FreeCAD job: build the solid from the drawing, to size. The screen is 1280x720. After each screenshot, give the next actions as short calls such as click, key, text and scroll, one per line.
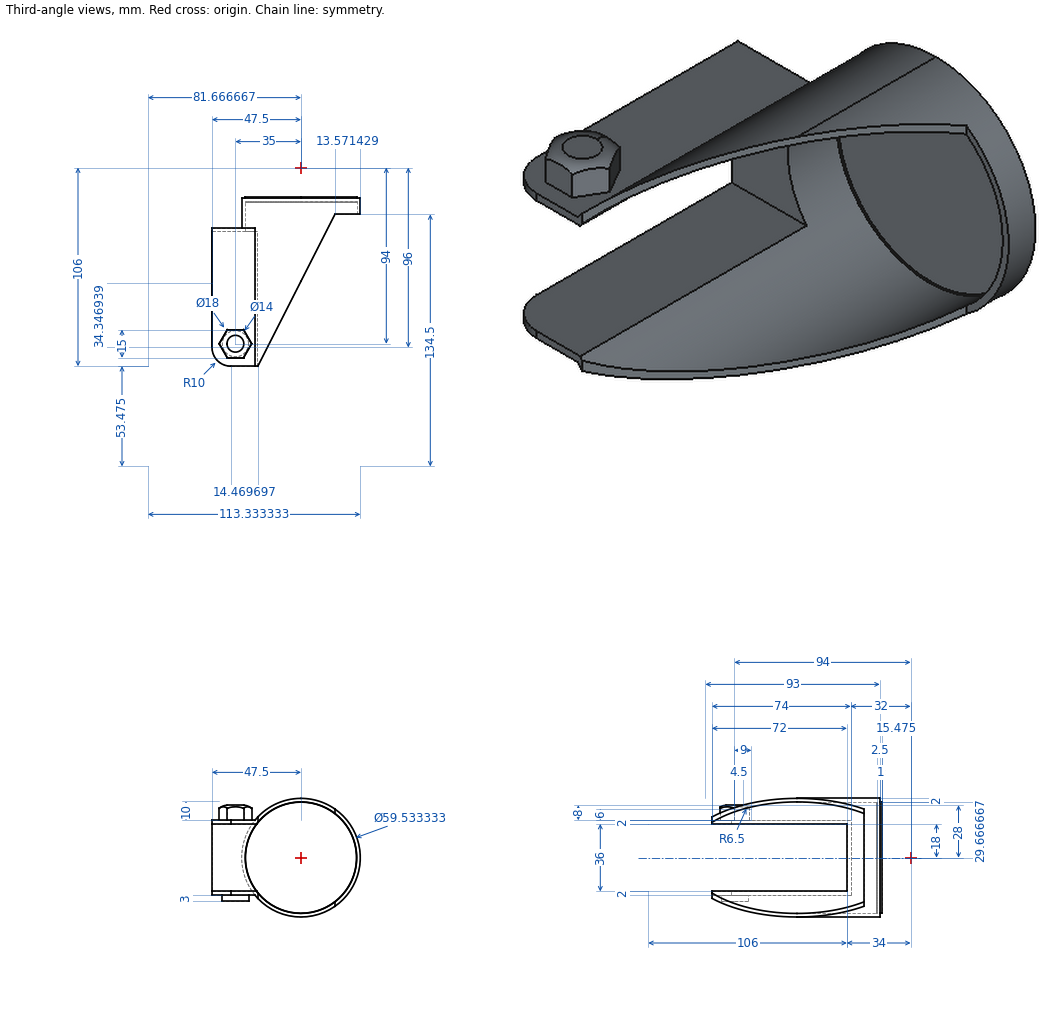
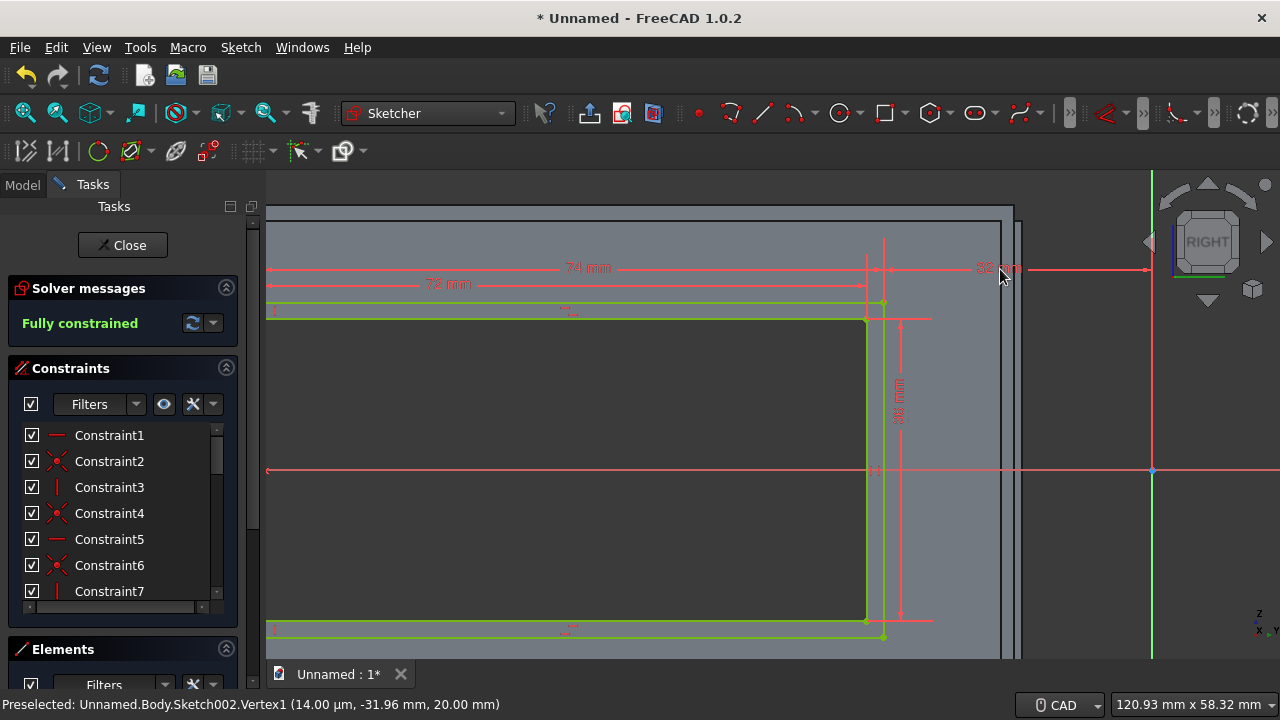
click(123, 245)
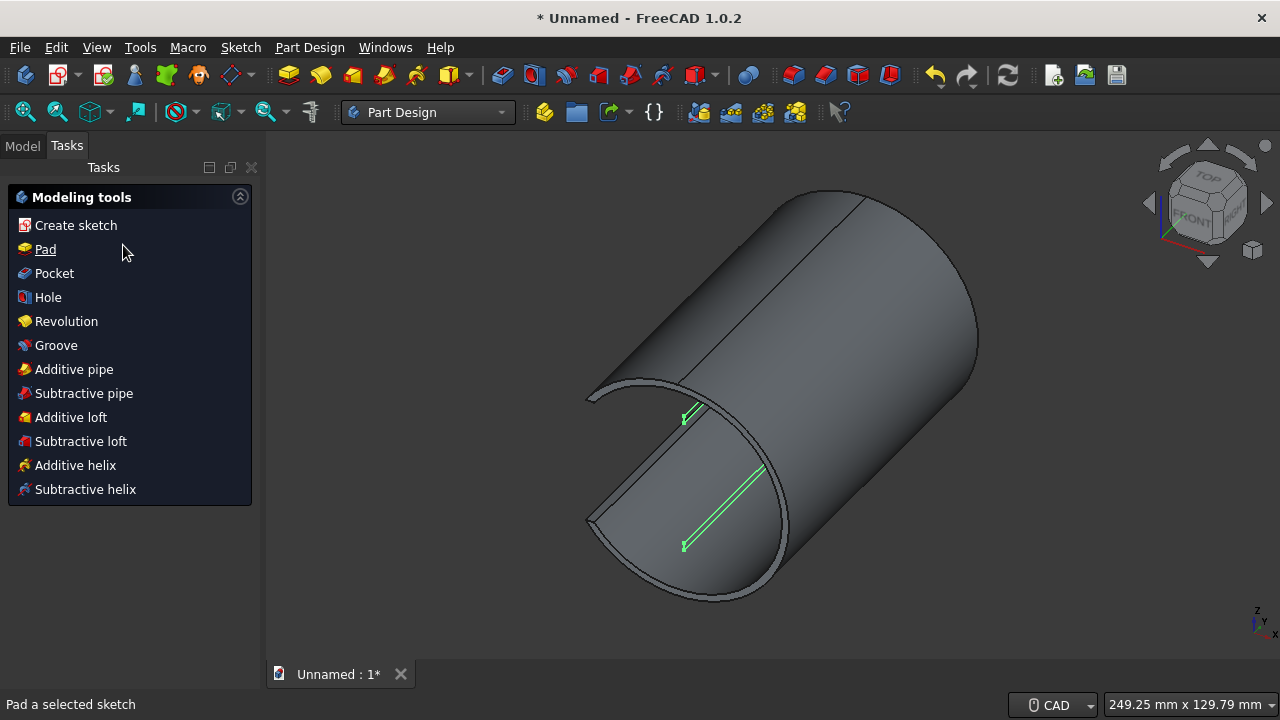
click(290, 76)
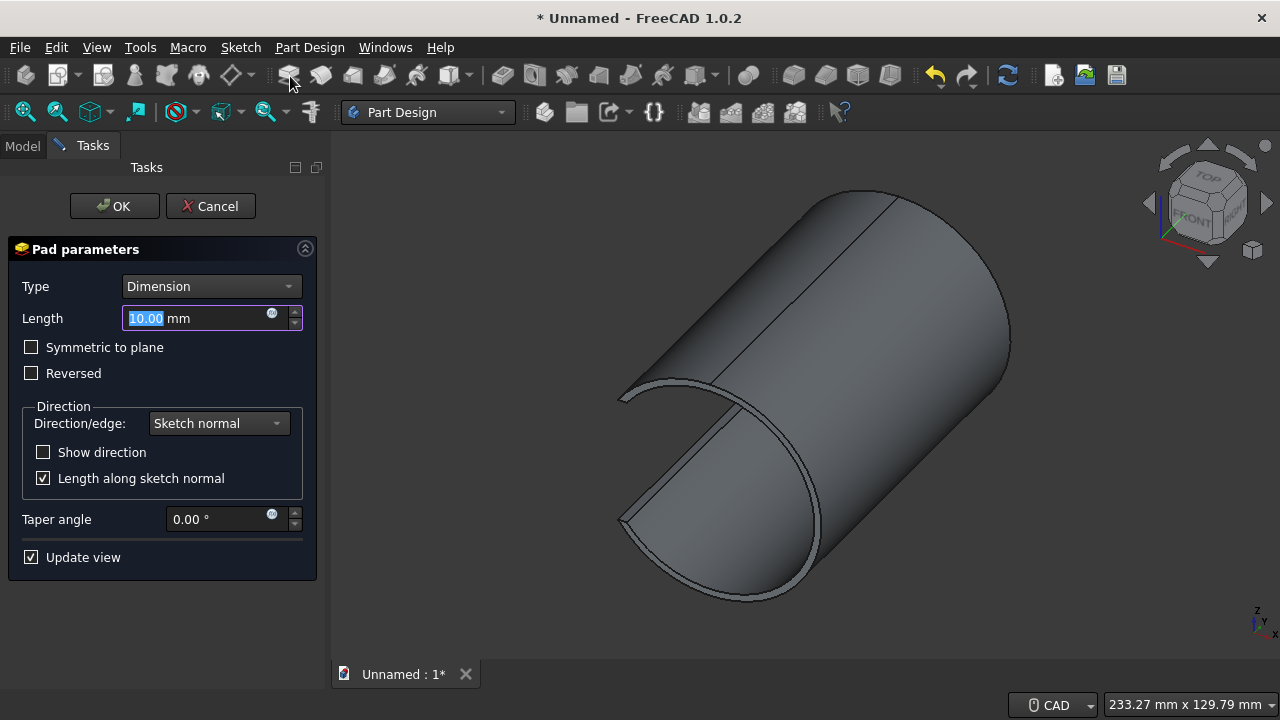
text(47.5)
key(Tab)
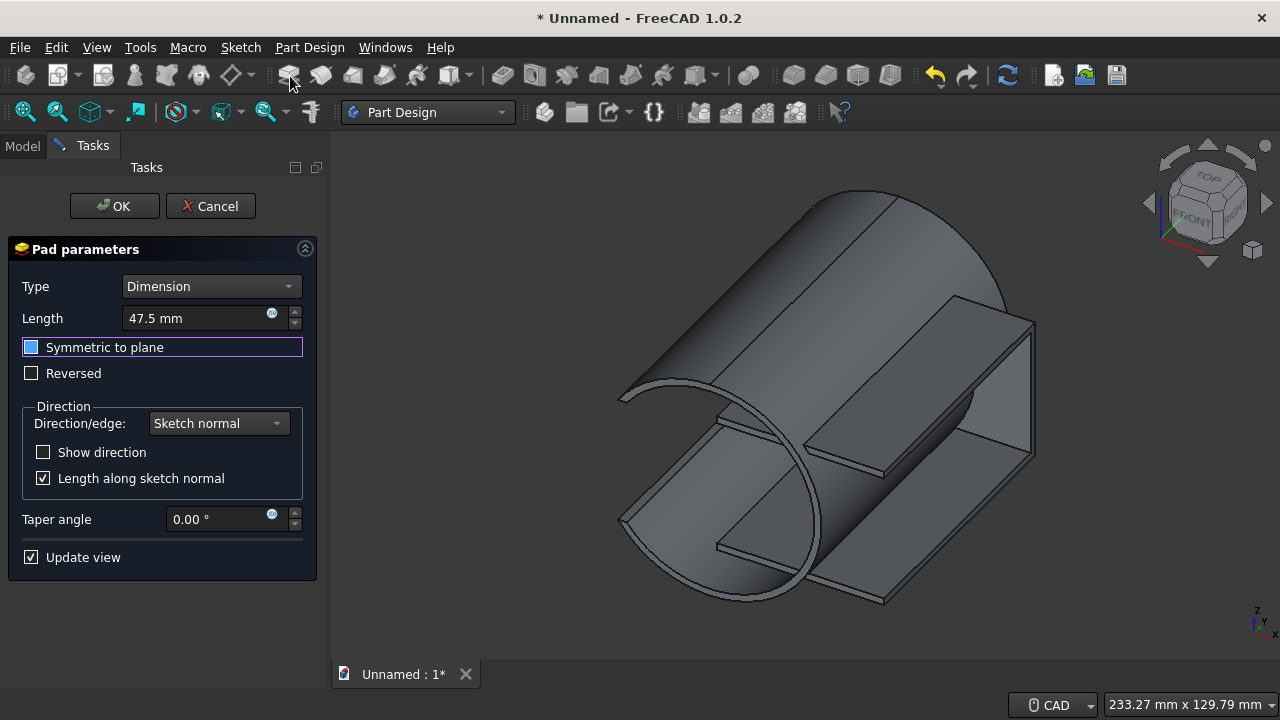
click(30, 373)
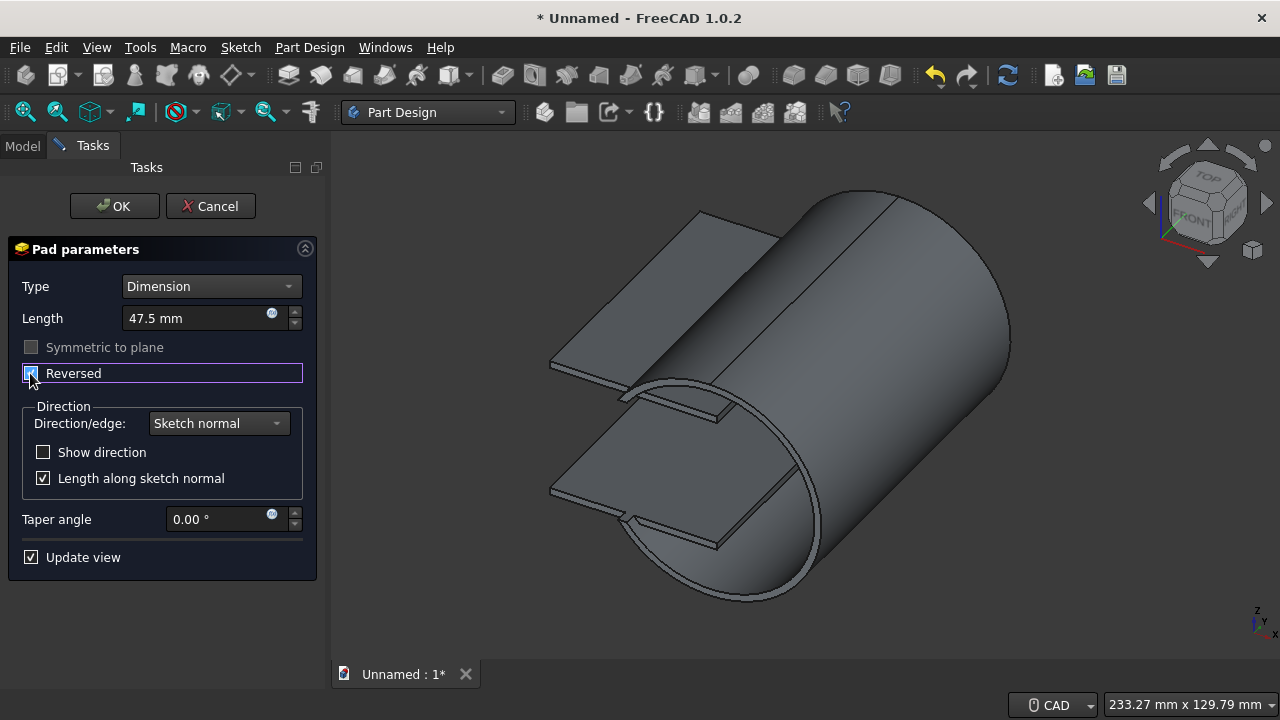
click(115, 206)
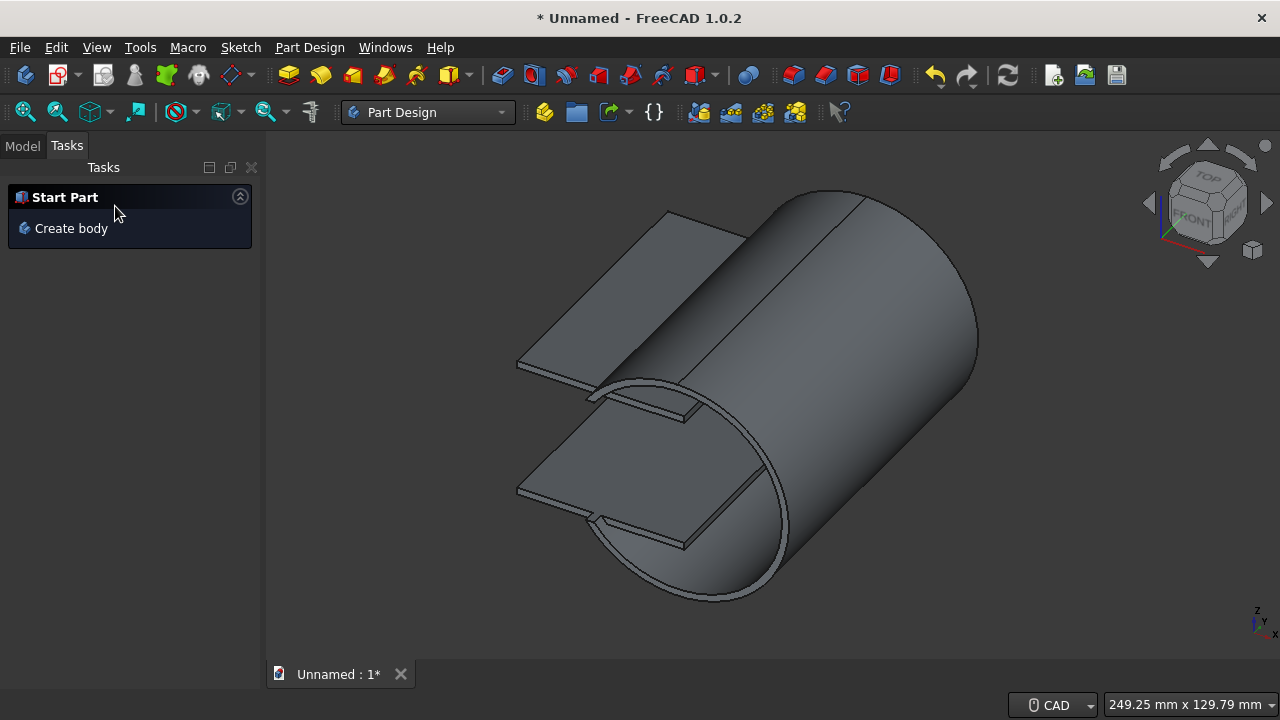
click(23, 145)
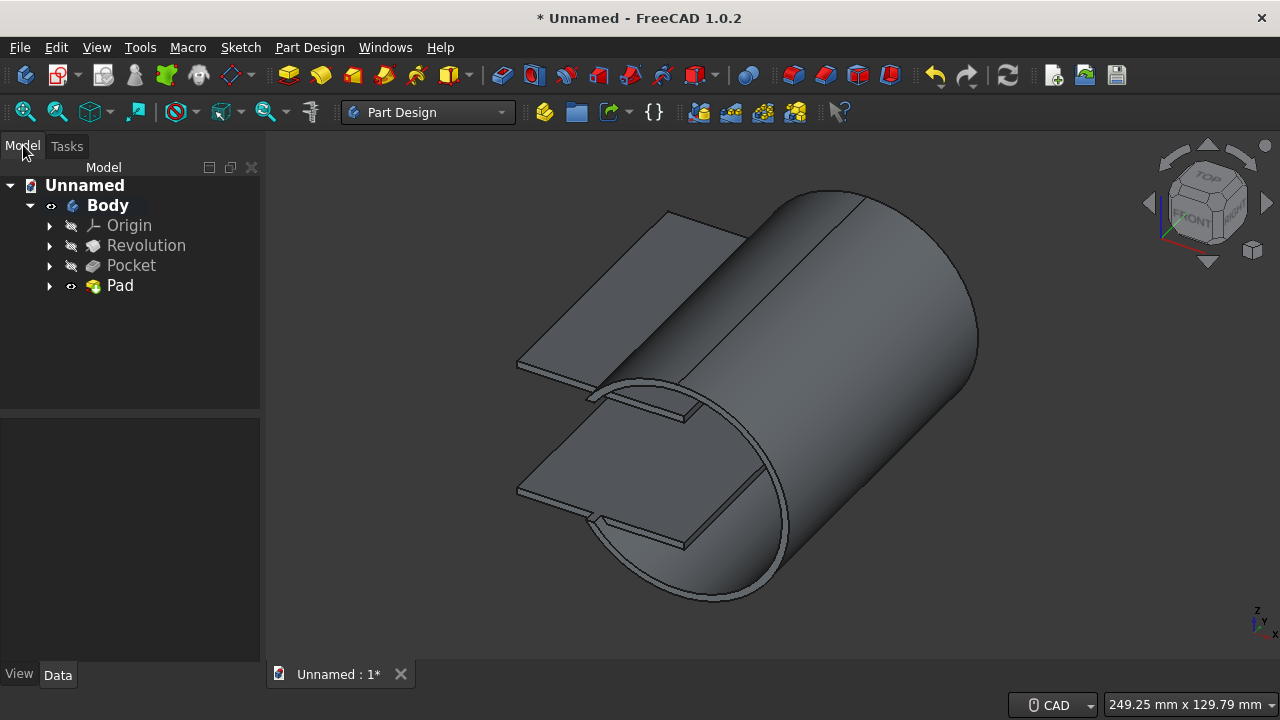
click(50, 226)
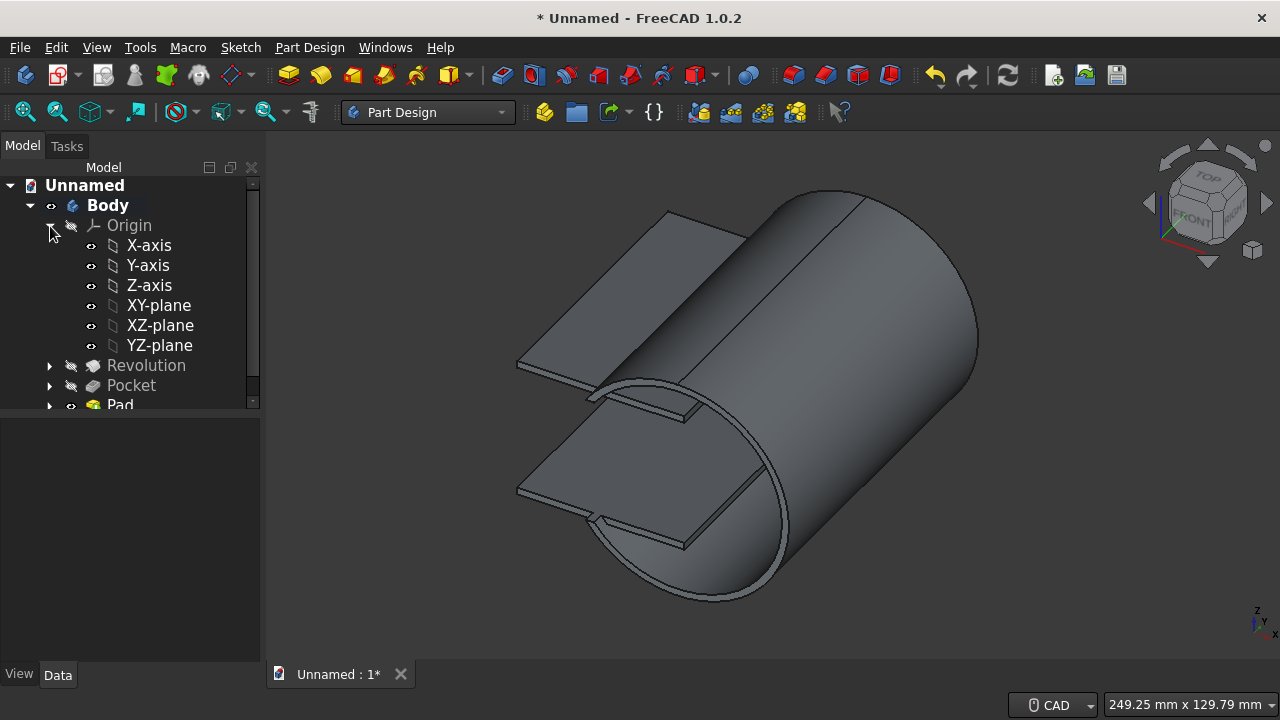
click(136, 326)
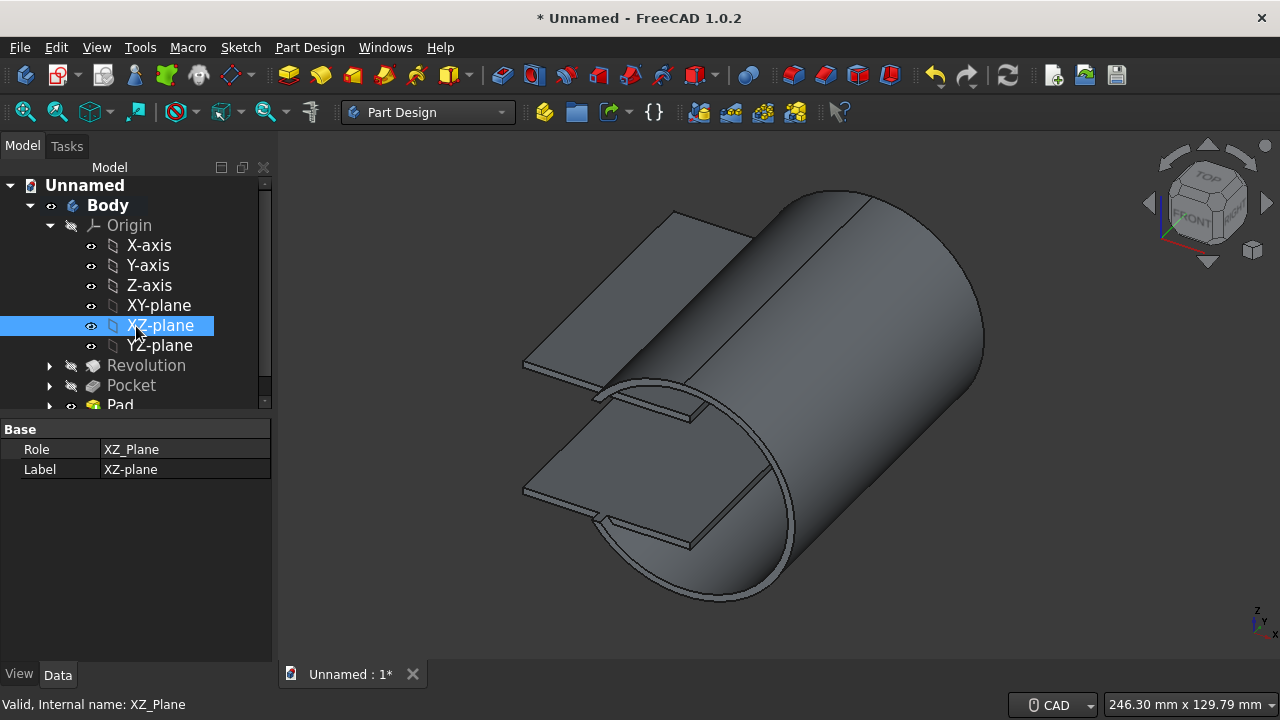
click(232, 76)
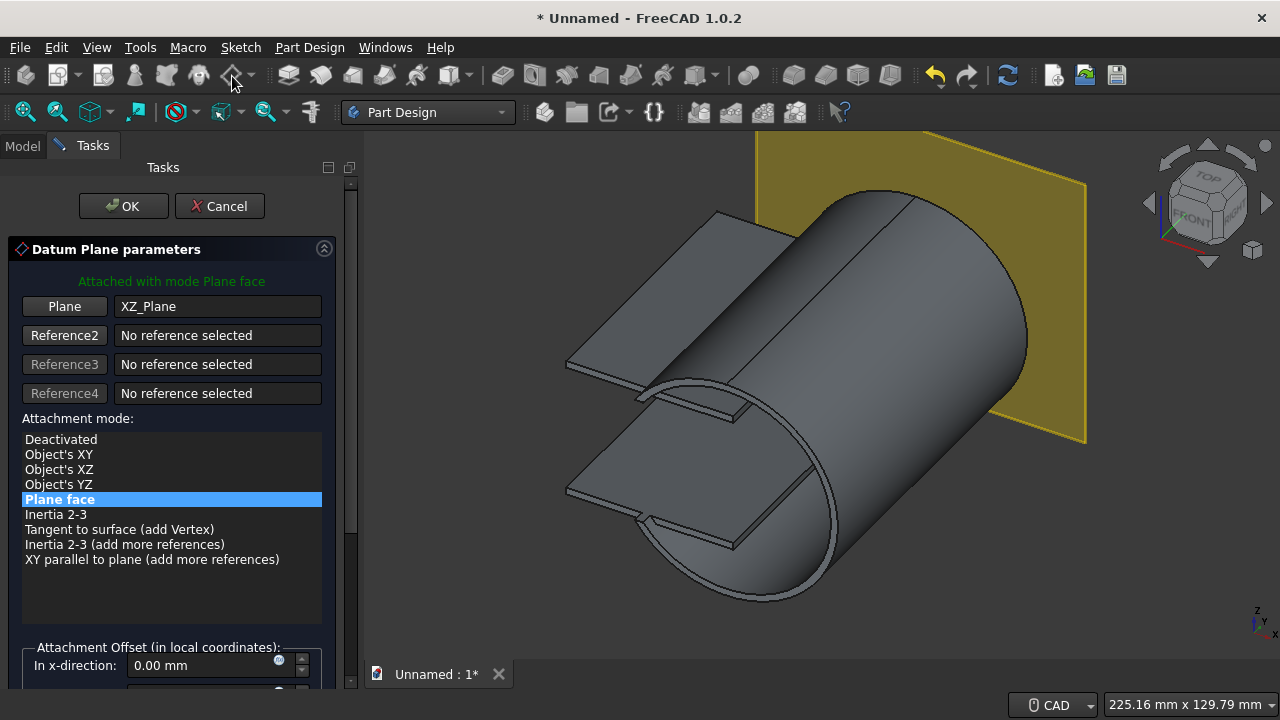
scroll(351, 432, down, 2)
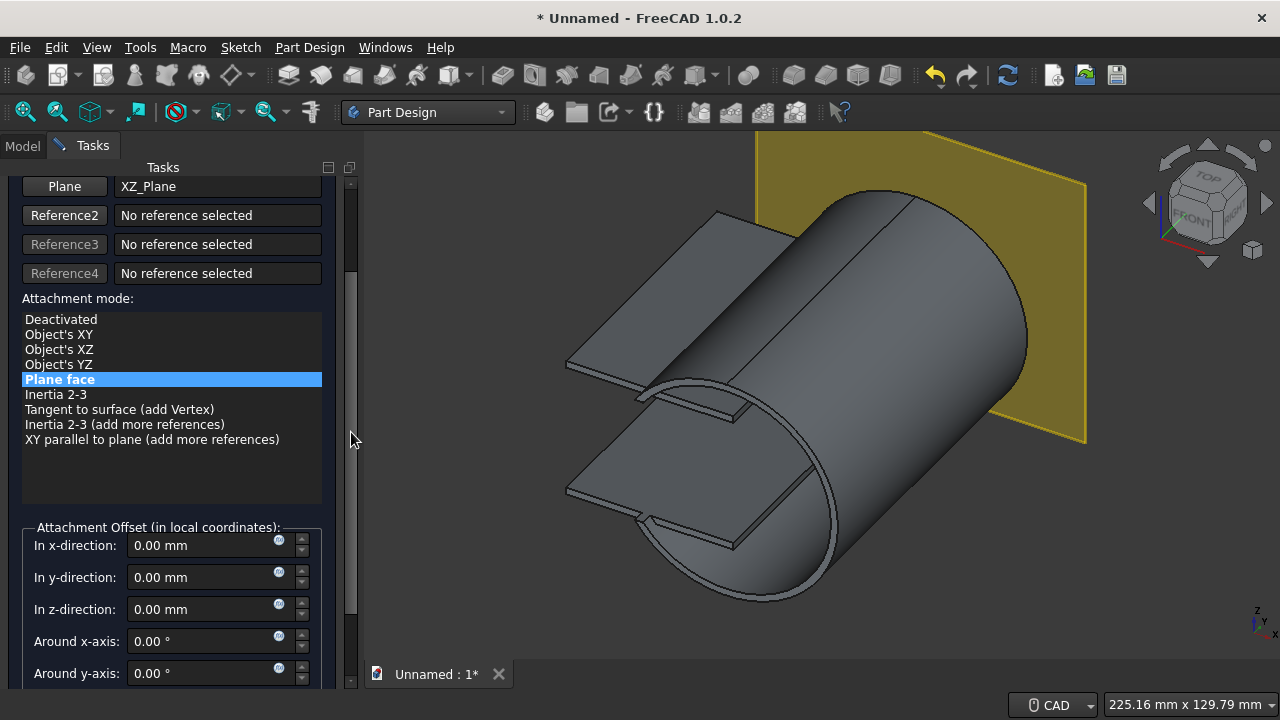
triple_click(210, 609)